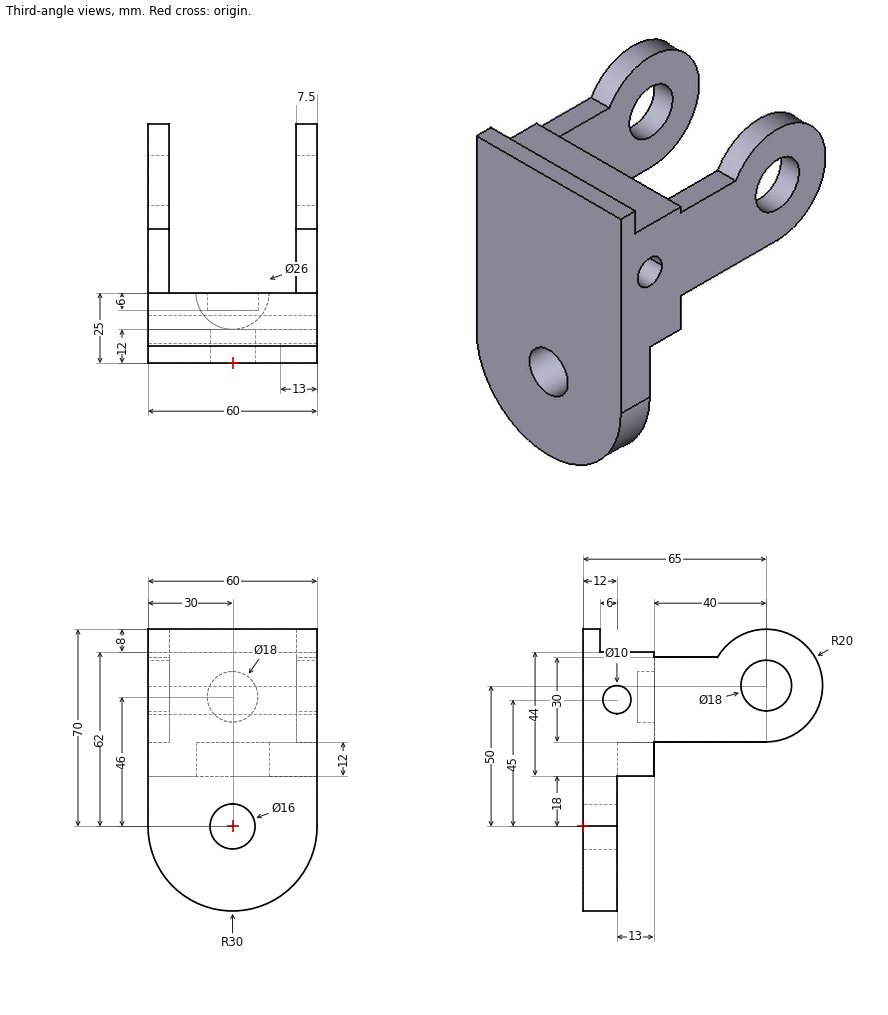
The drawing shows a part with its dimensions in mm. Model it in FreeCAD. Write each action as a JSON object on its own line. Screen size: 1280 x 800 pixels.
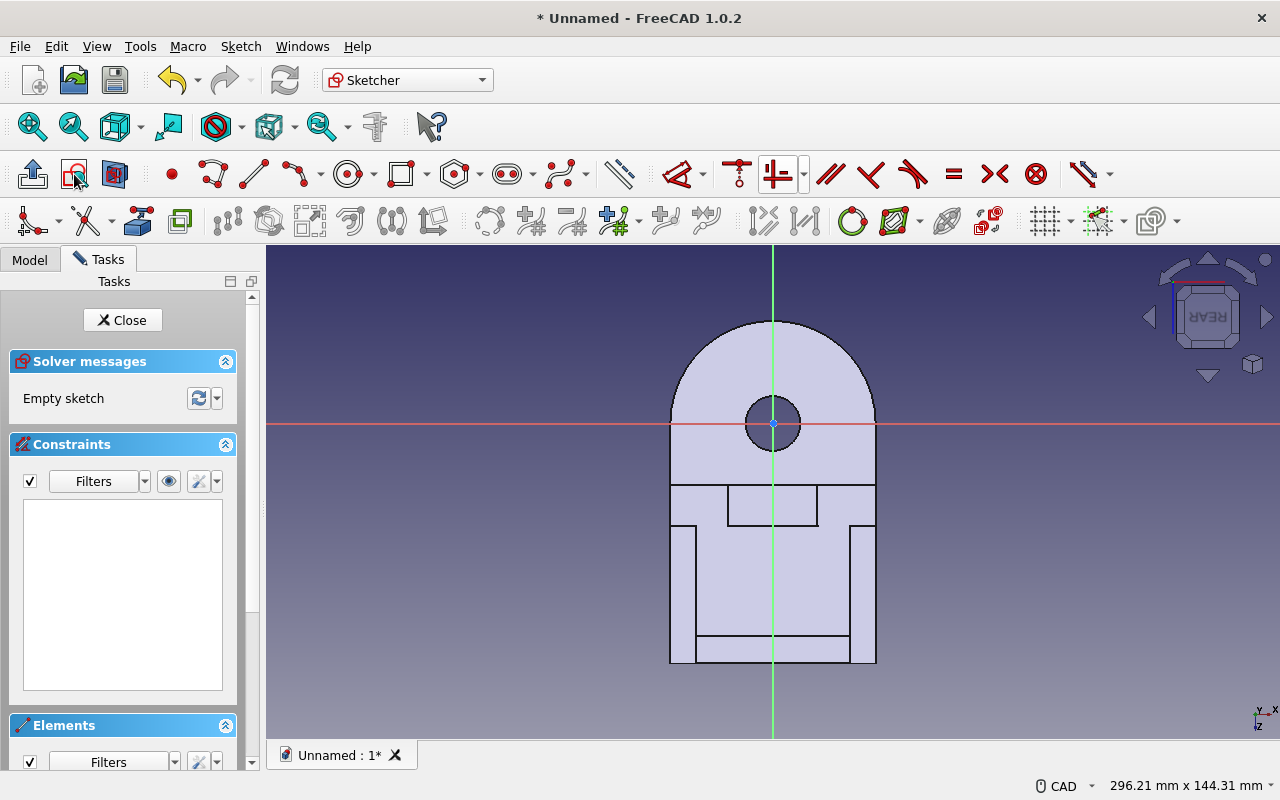
{"action": "left_click", "coordinate": [115, 174]}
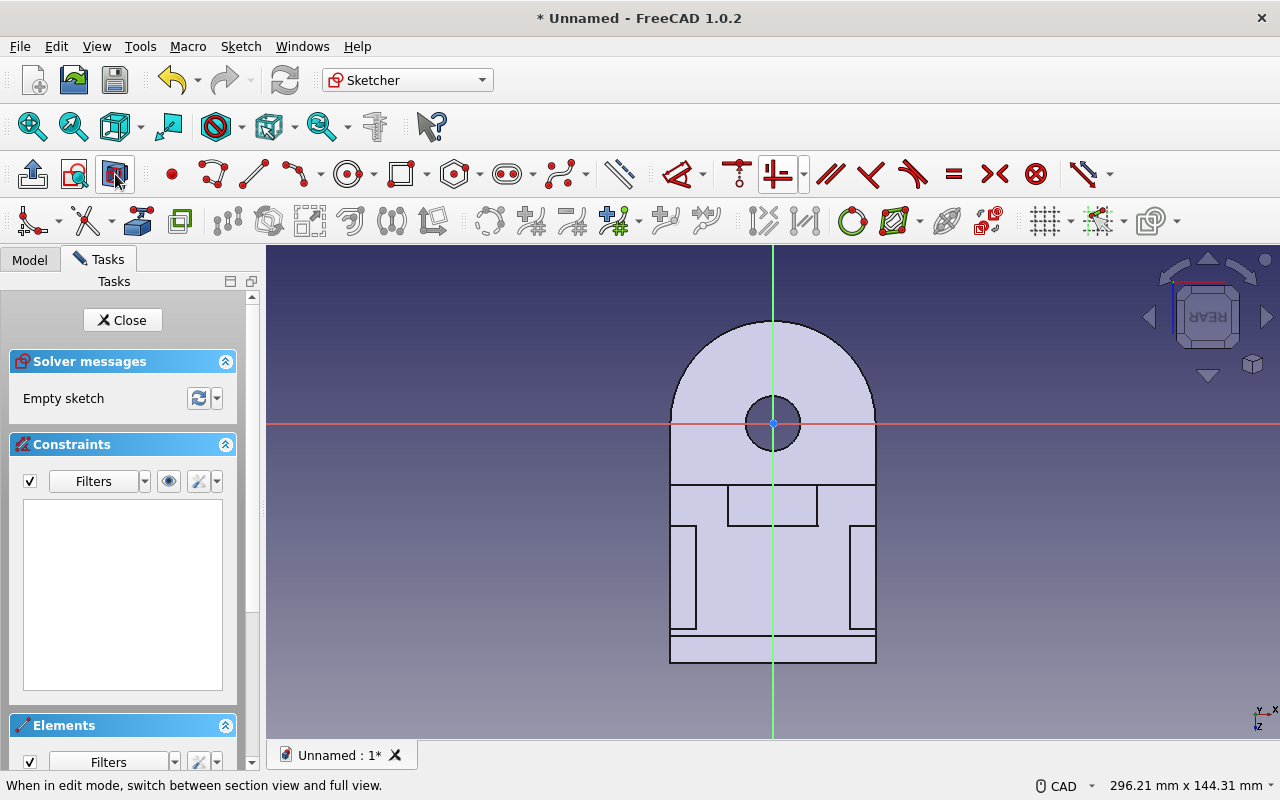
{"action": "scroll", "coordinate": [790, 604], "scroll_direction": "up", "scroll_amount": 8}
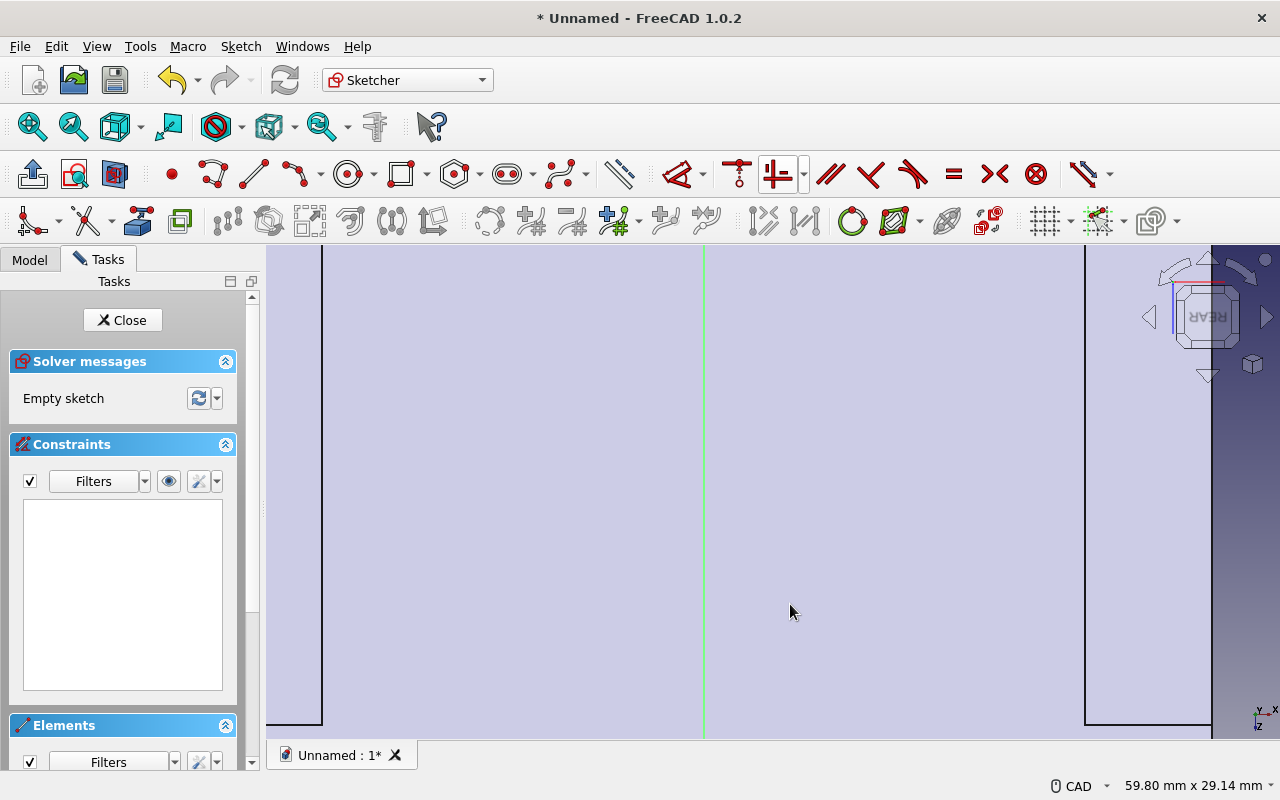
{"action": "key", "text": "g c"}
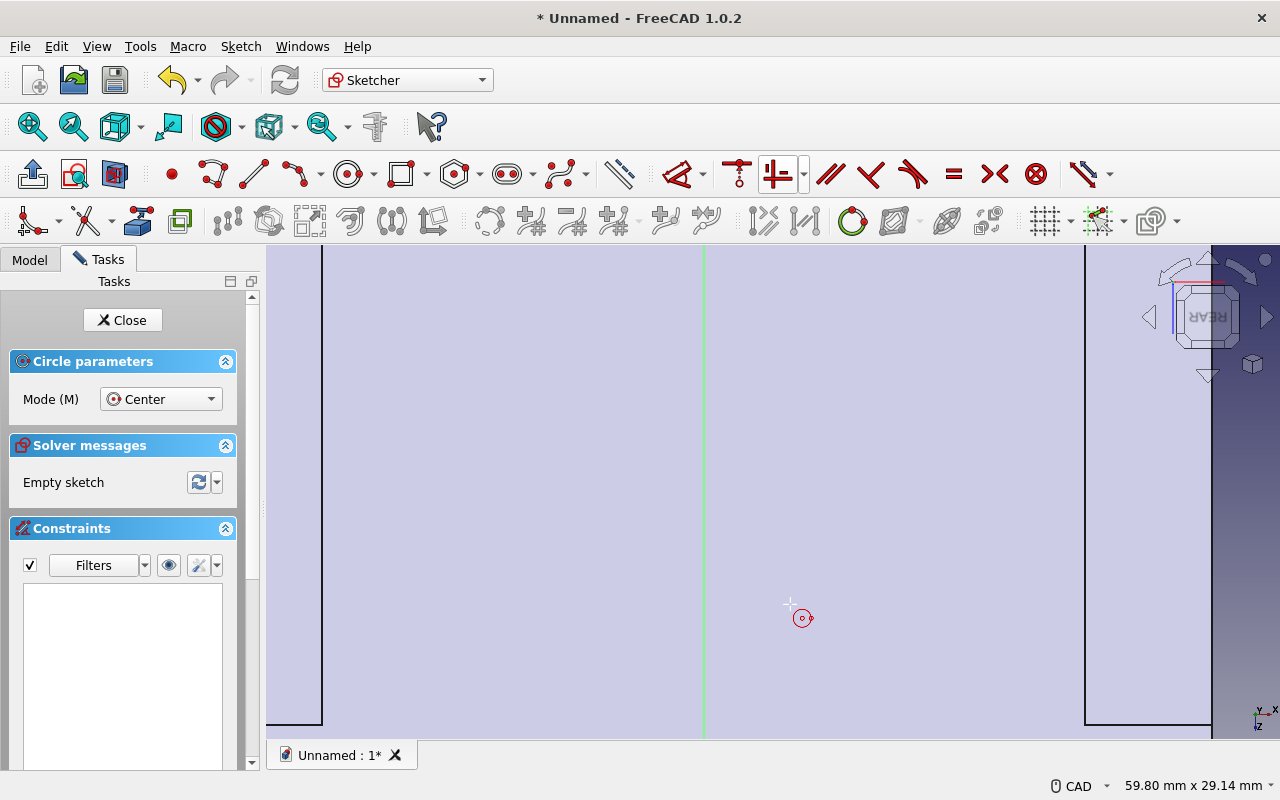
{"action": "left_click", "coordinate": [704, 487]}
{"action": "left_click", "coordinate": [812, 379]}
{"action": "key", "text": "Escape"}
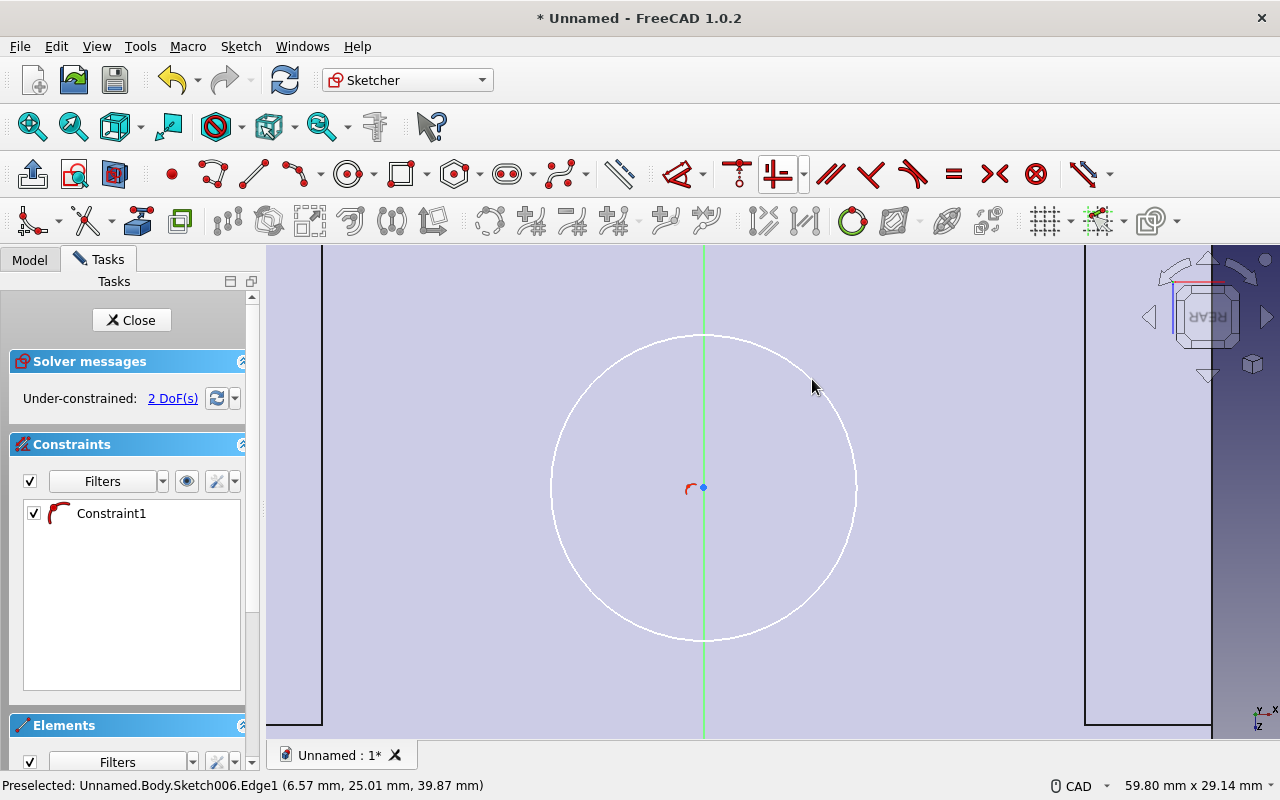
{"action": "key", "text": "d"}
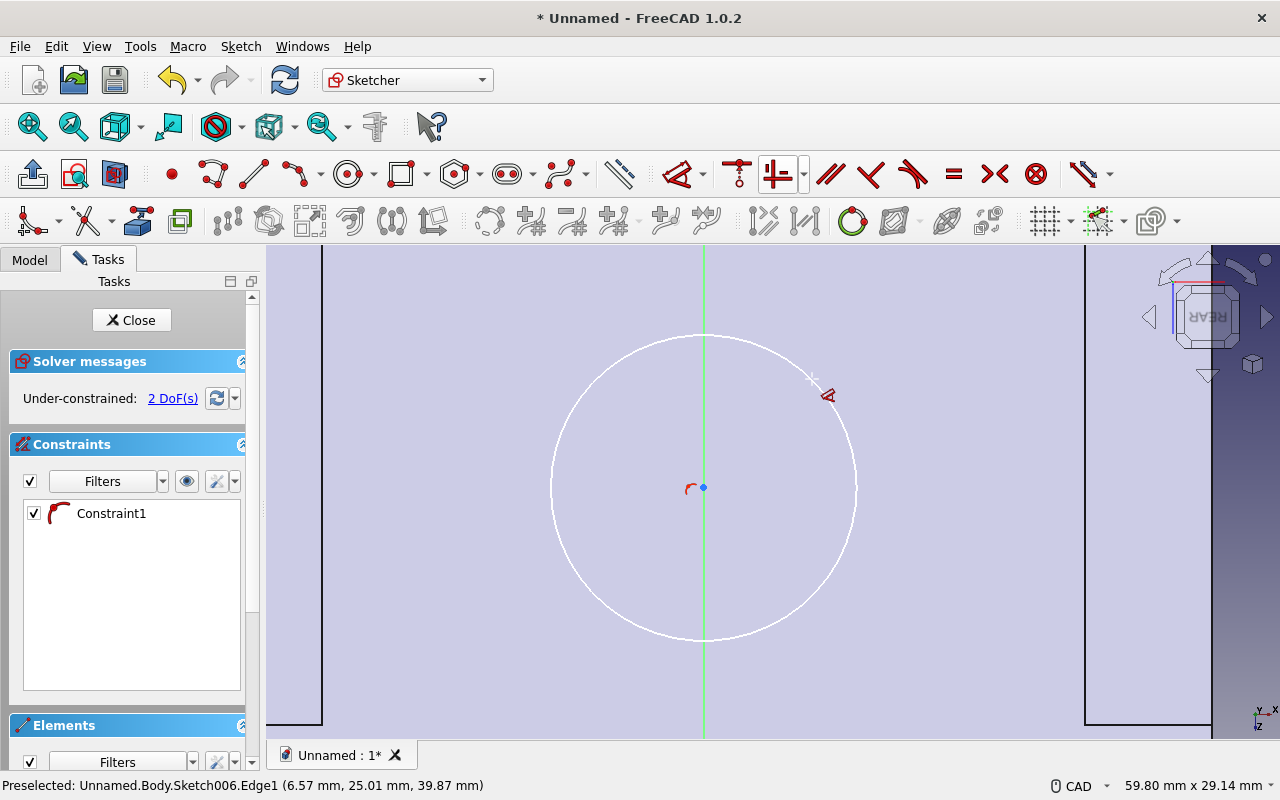
{"action": "left_click", "coordinate": [812, 380]}
{"action": "left_click", "coordinate": [835, 357]}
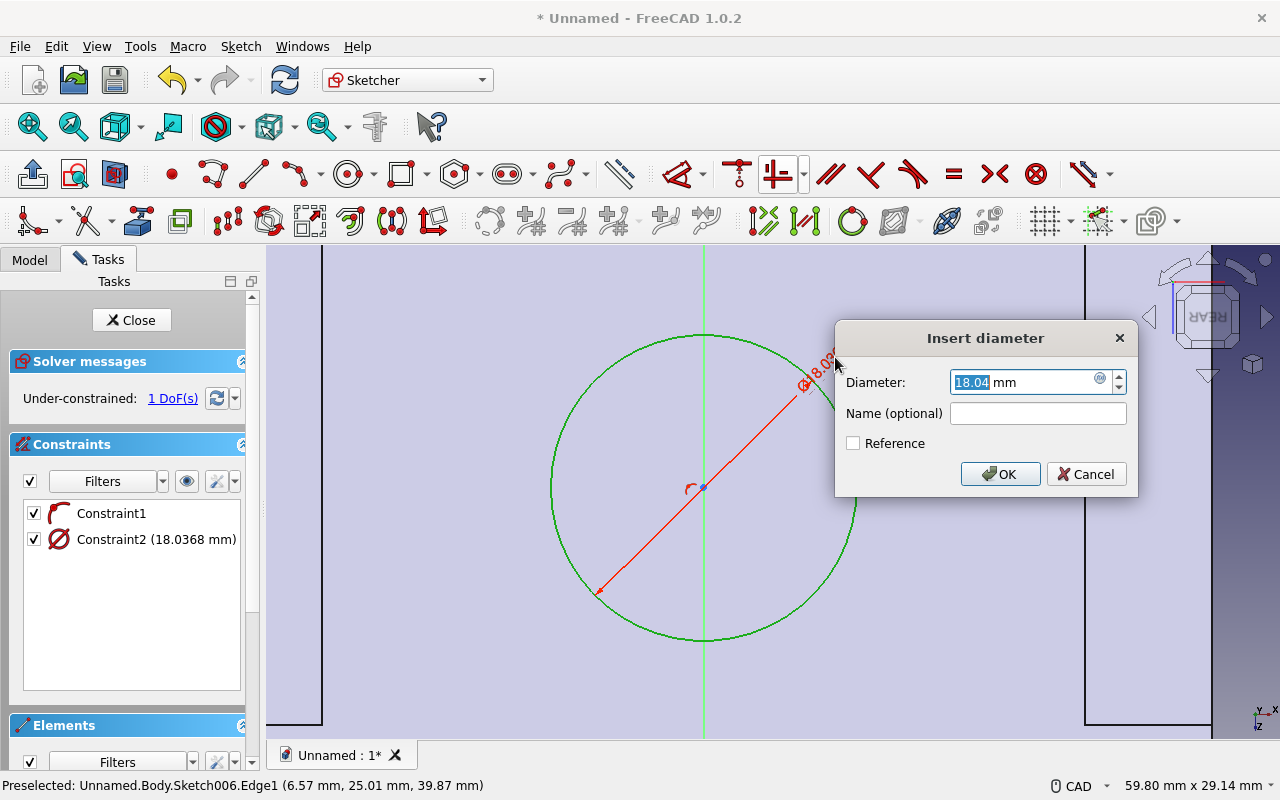
{"action": "type", "text": "18"}
{"action": "key", "text": "Return"}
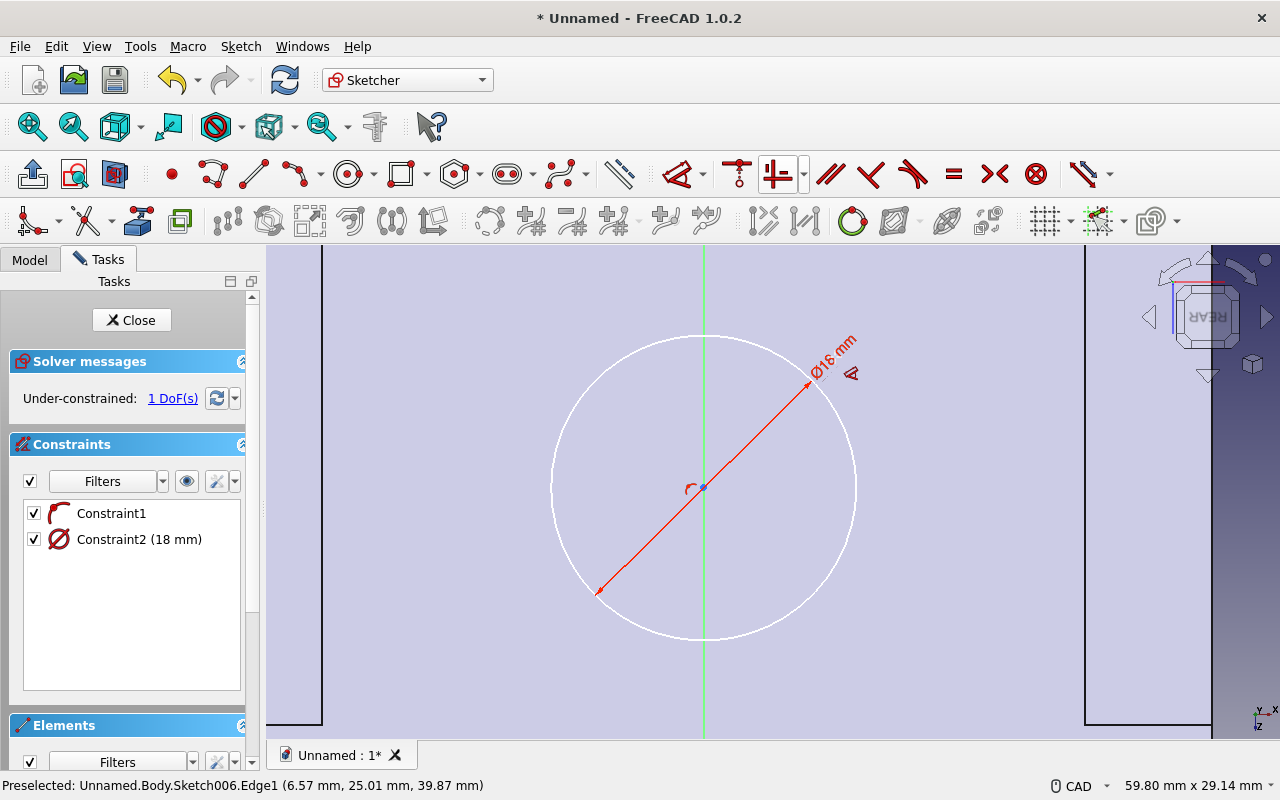
{"action": "left_click", "coordinate": [704, 488]}
{"action": "left_click", "coordinate": [738, 380]}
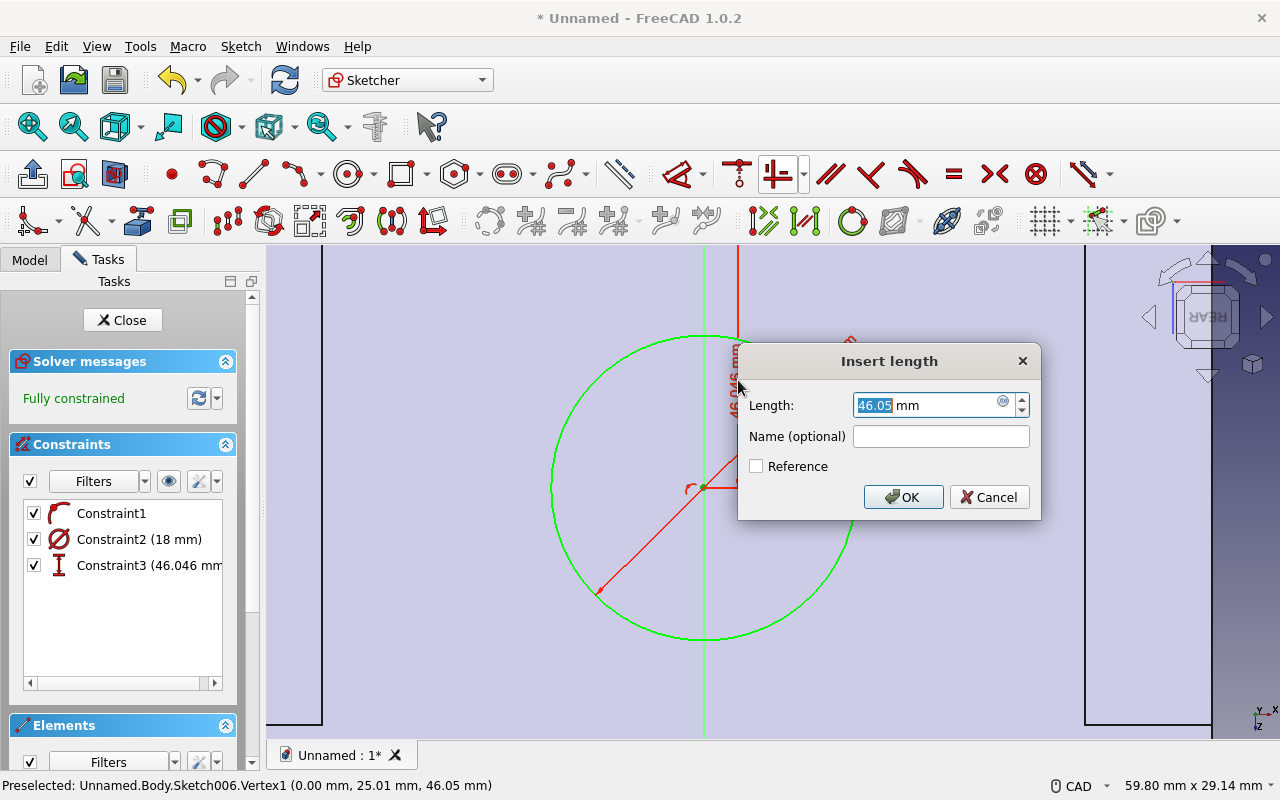
{"action": "type", "text": "46"}
{"action": "key", "text": "Return"}
{"action": "key", "text": "Escape"}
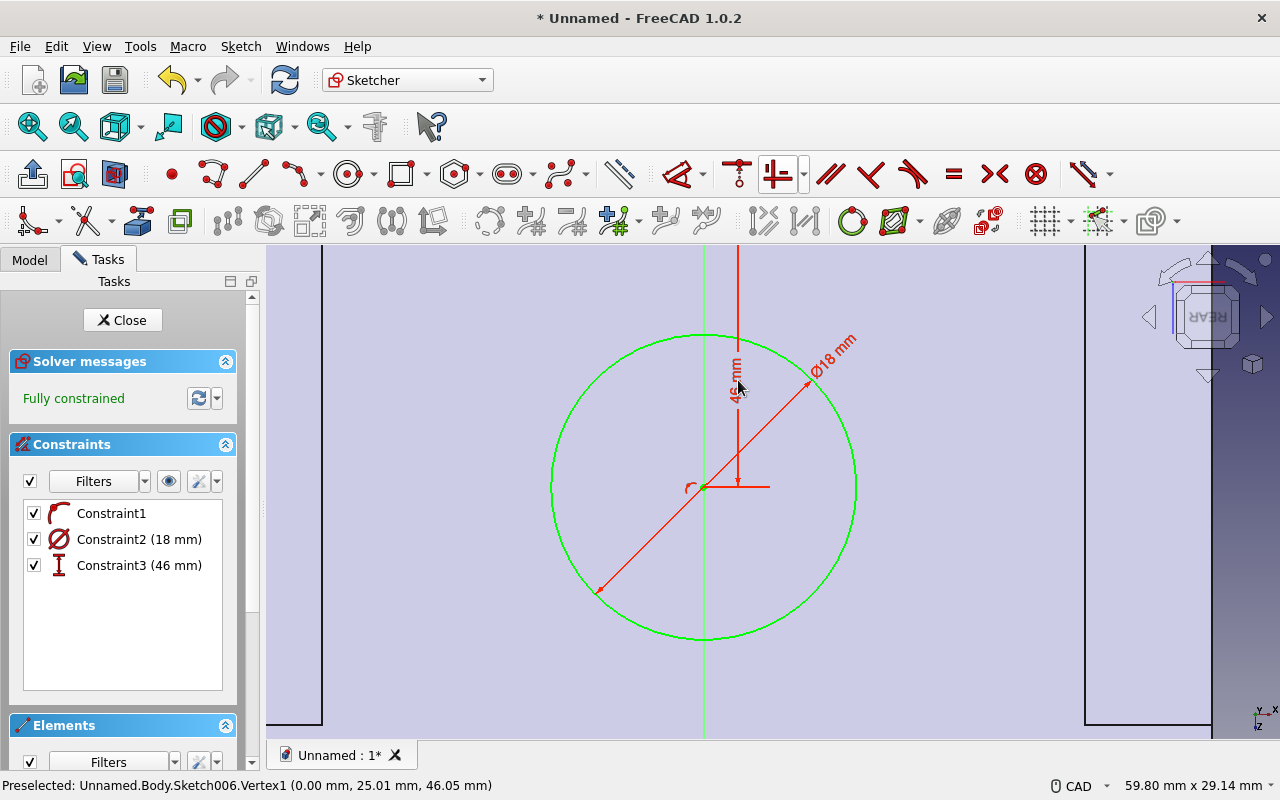
{"action": "left_click", "coordinate": [123, 320]}